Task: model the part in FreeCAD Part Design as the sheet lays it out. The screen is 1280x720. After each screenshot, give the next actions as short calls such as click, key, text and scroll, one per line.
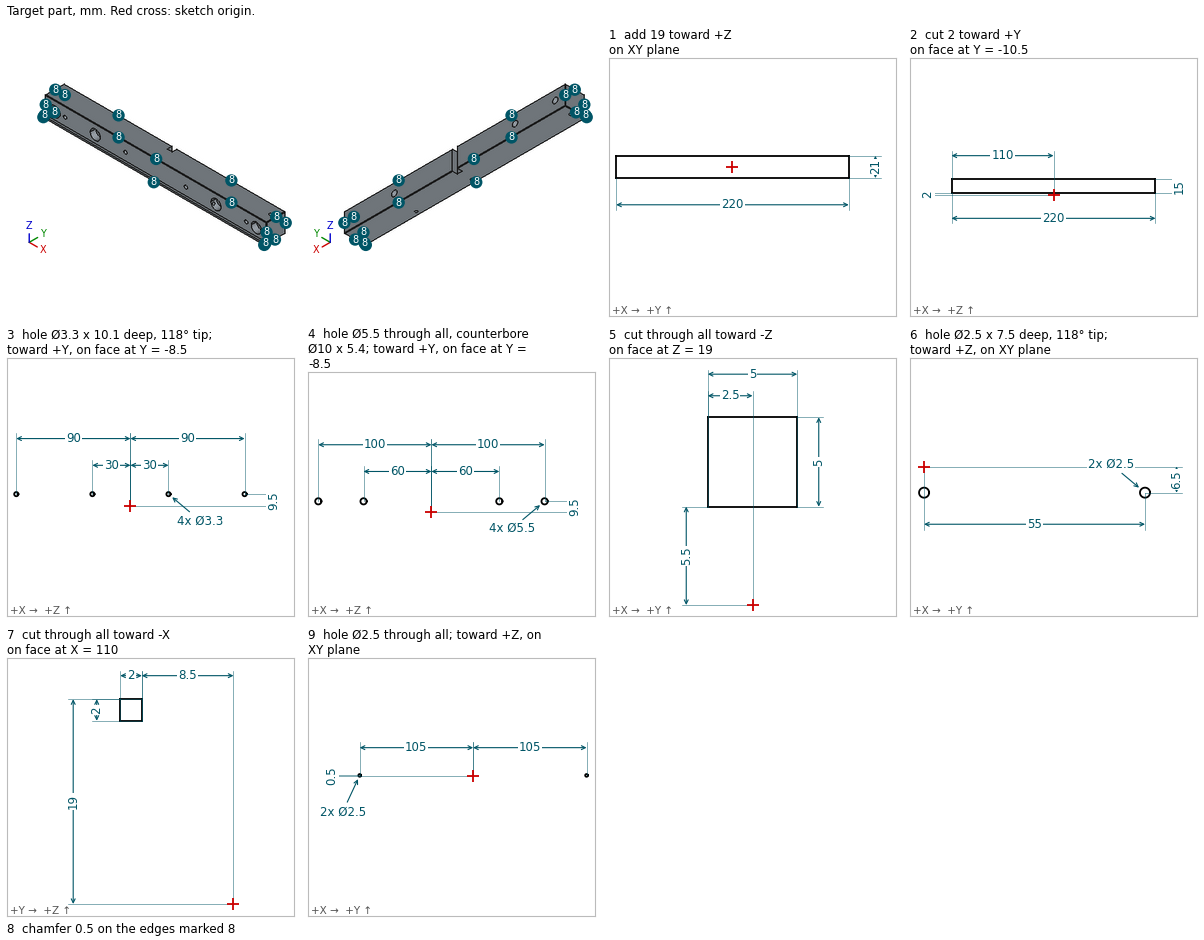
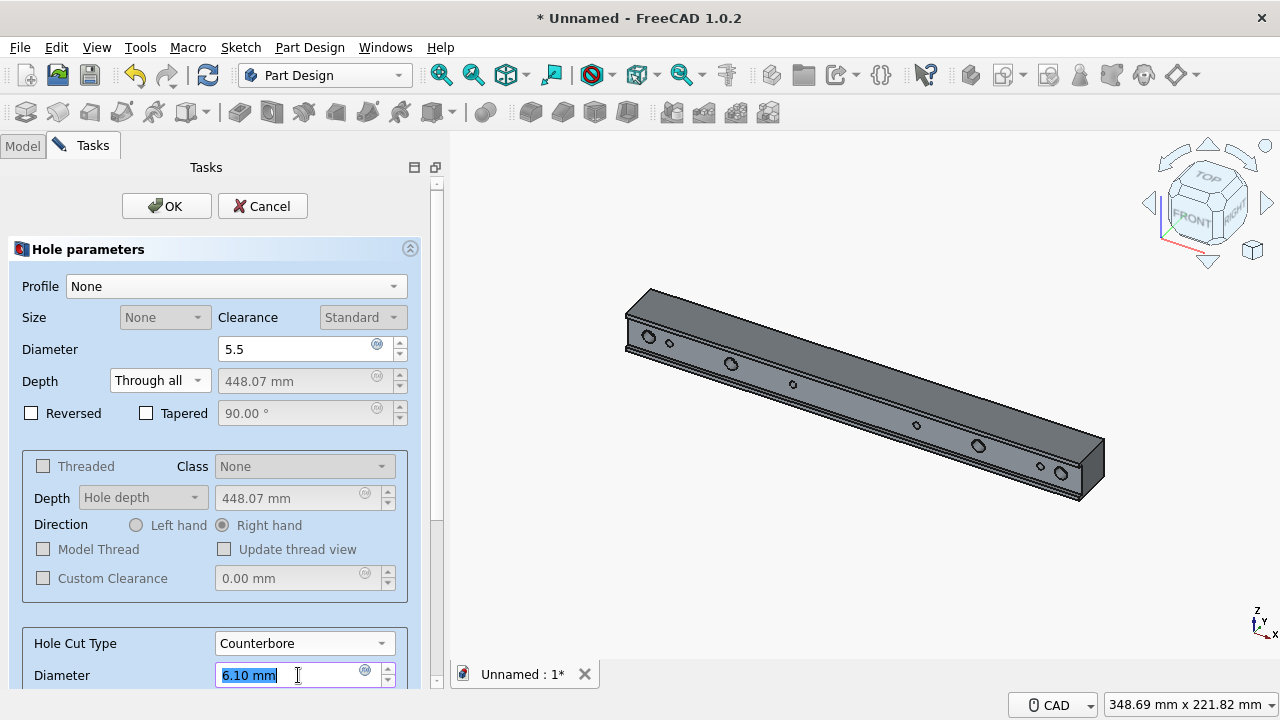
text(10)
key(Tab)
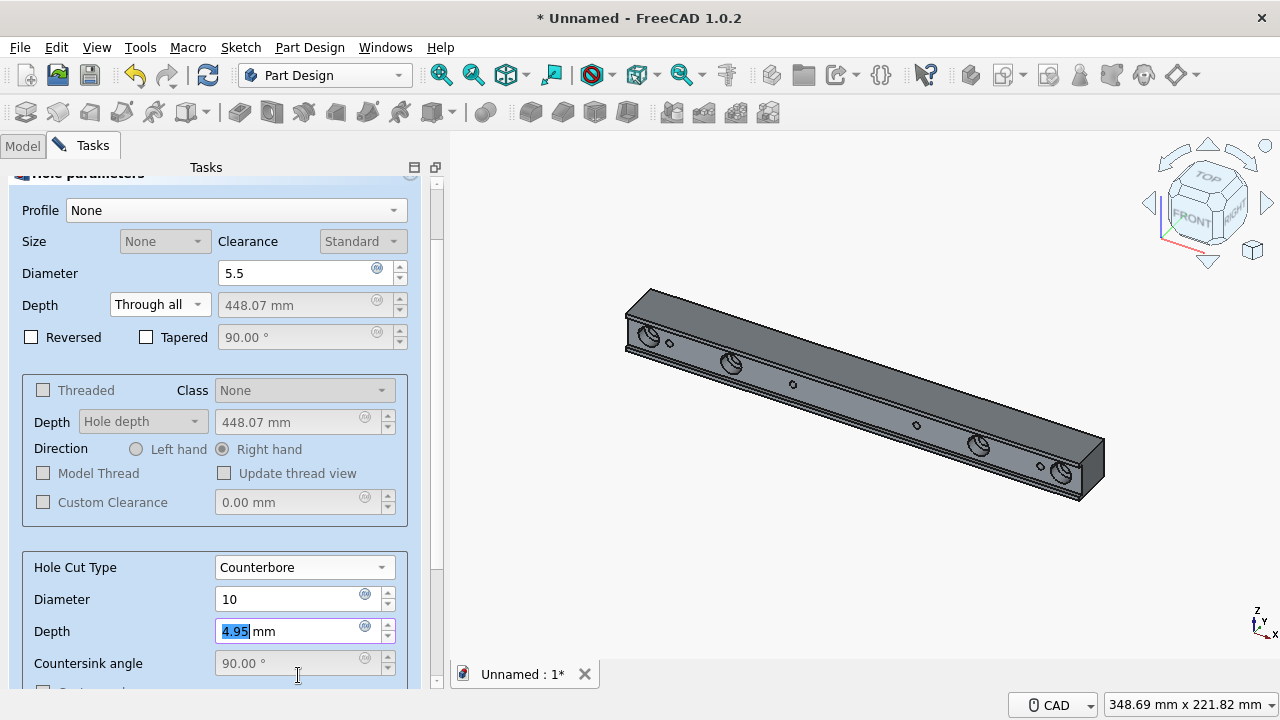
text(5.4)
key(Tab)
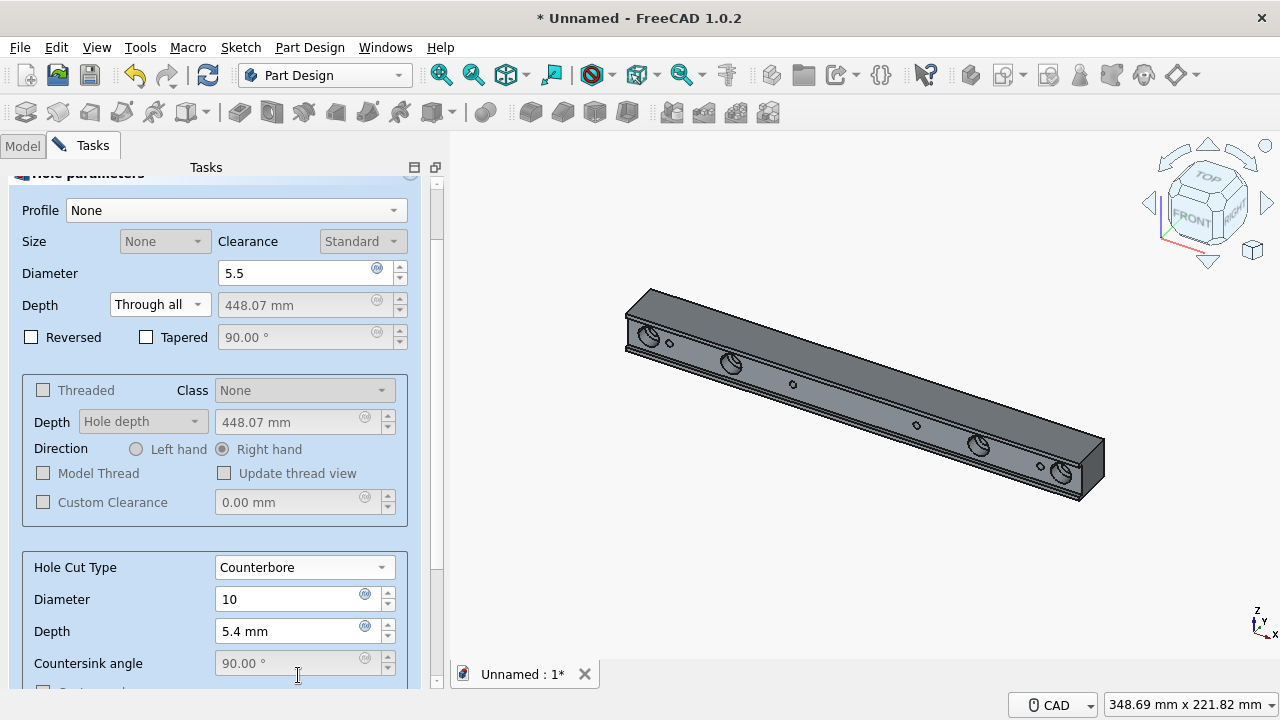
scroll(437, 432, up, 3)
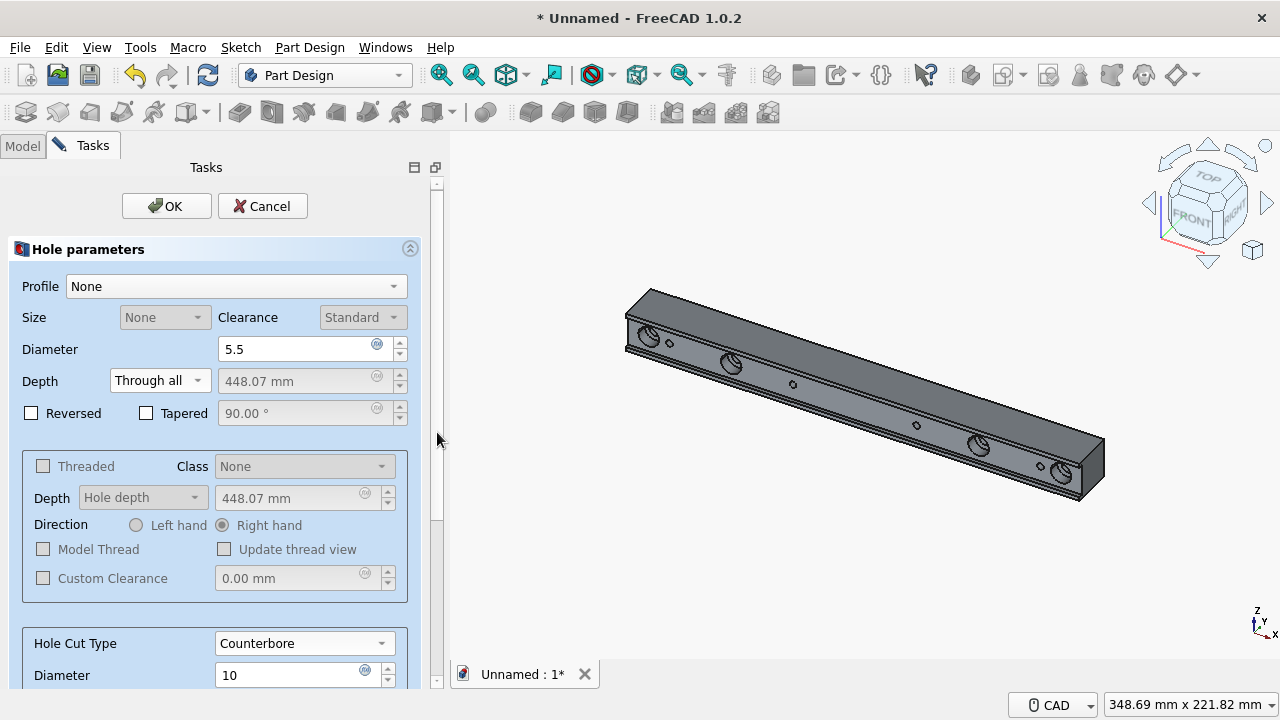
click(167, 206)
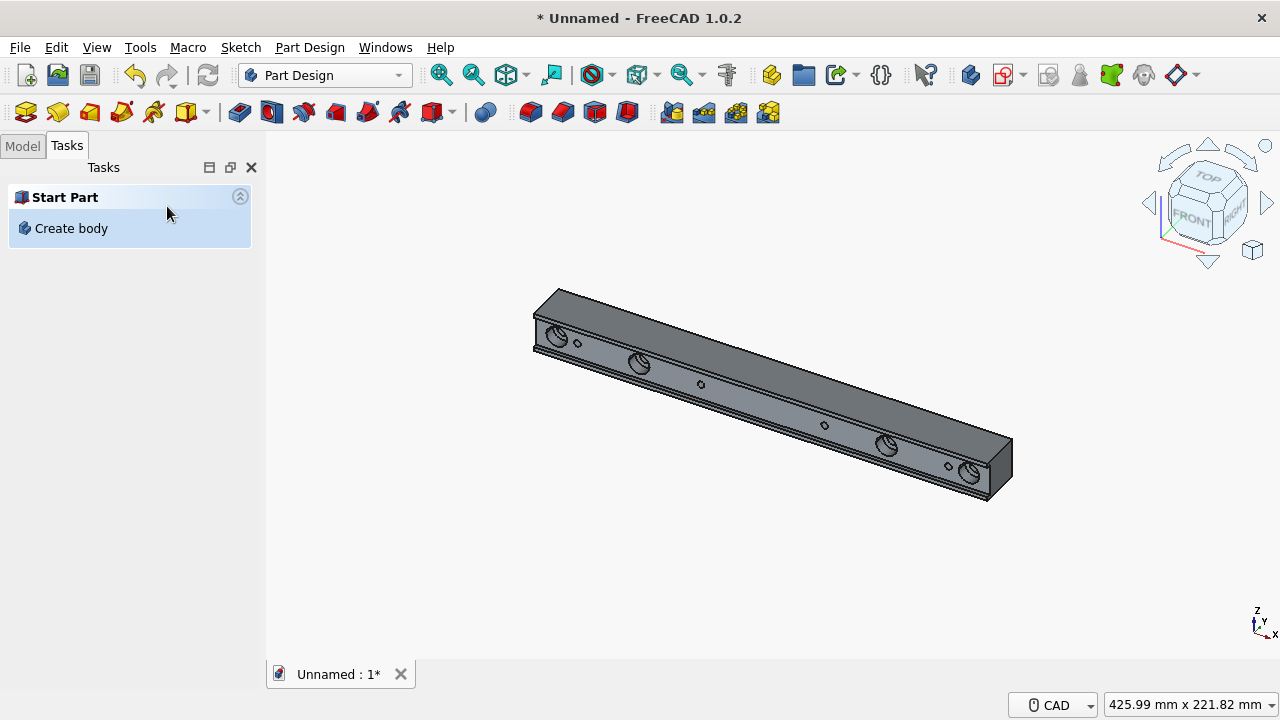
click(967, 440)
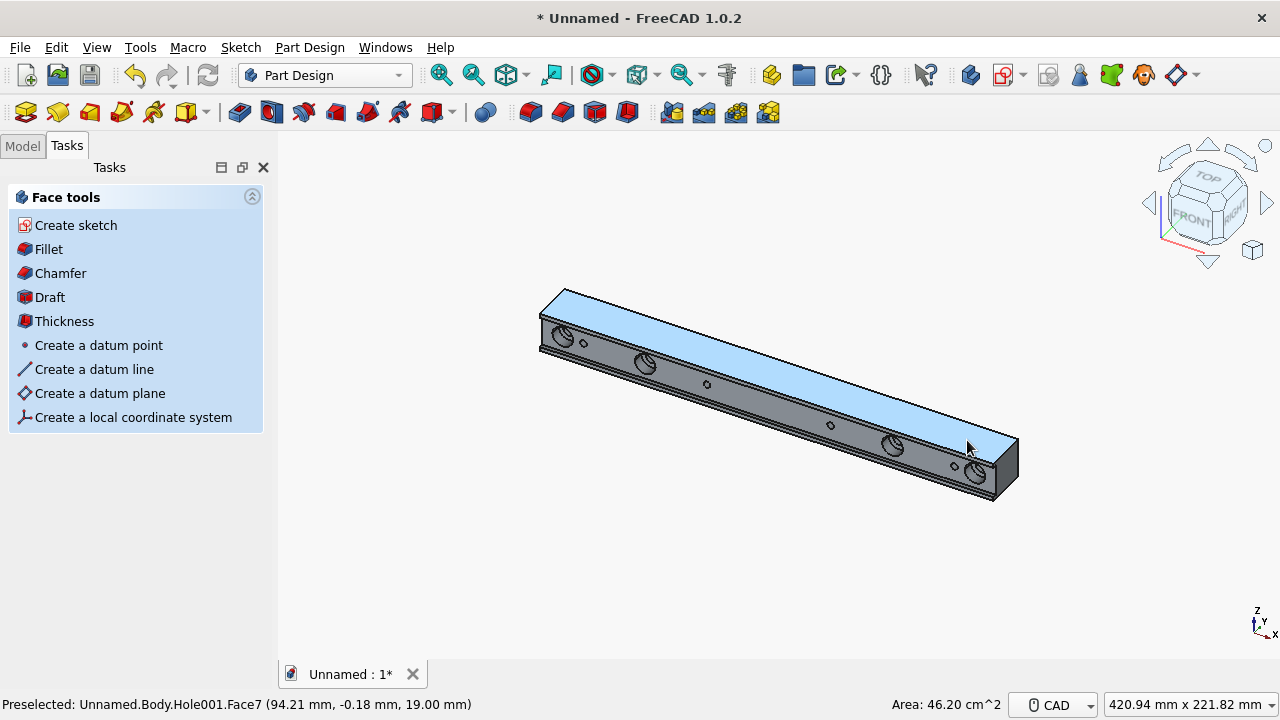
click(1004, 76)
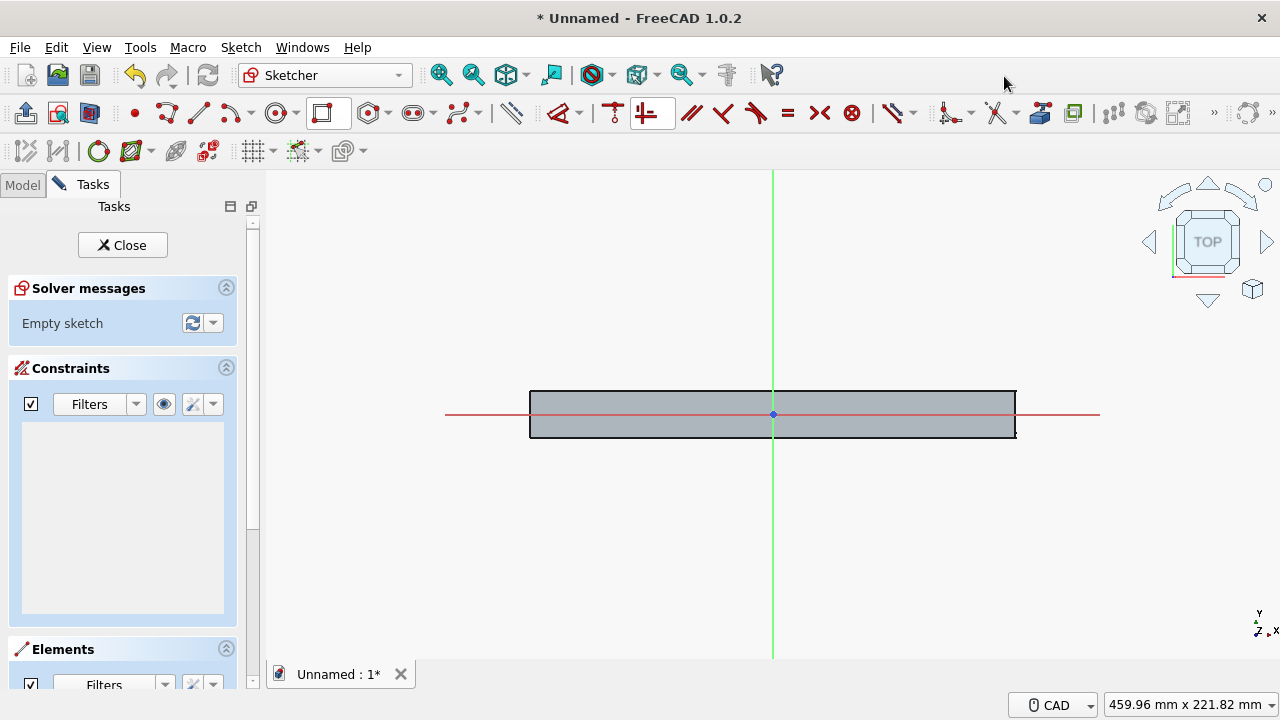
scroll(778, 402, up, 13)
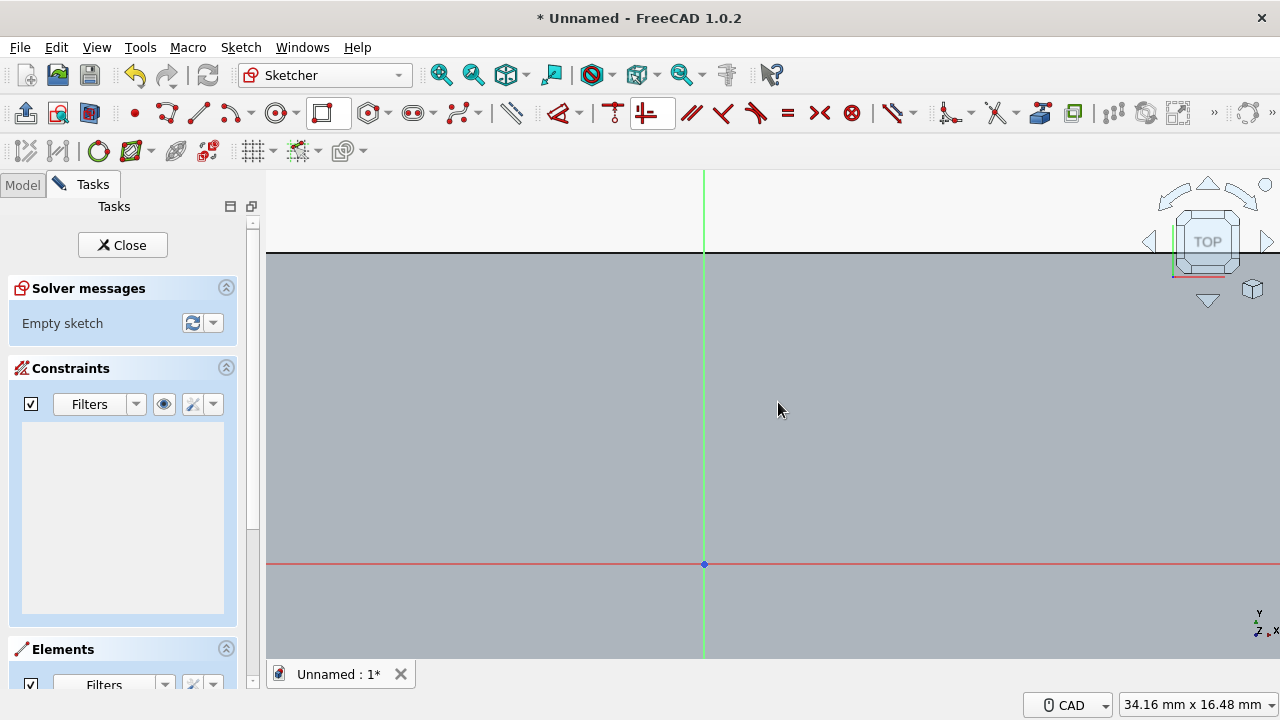
click(322, 114)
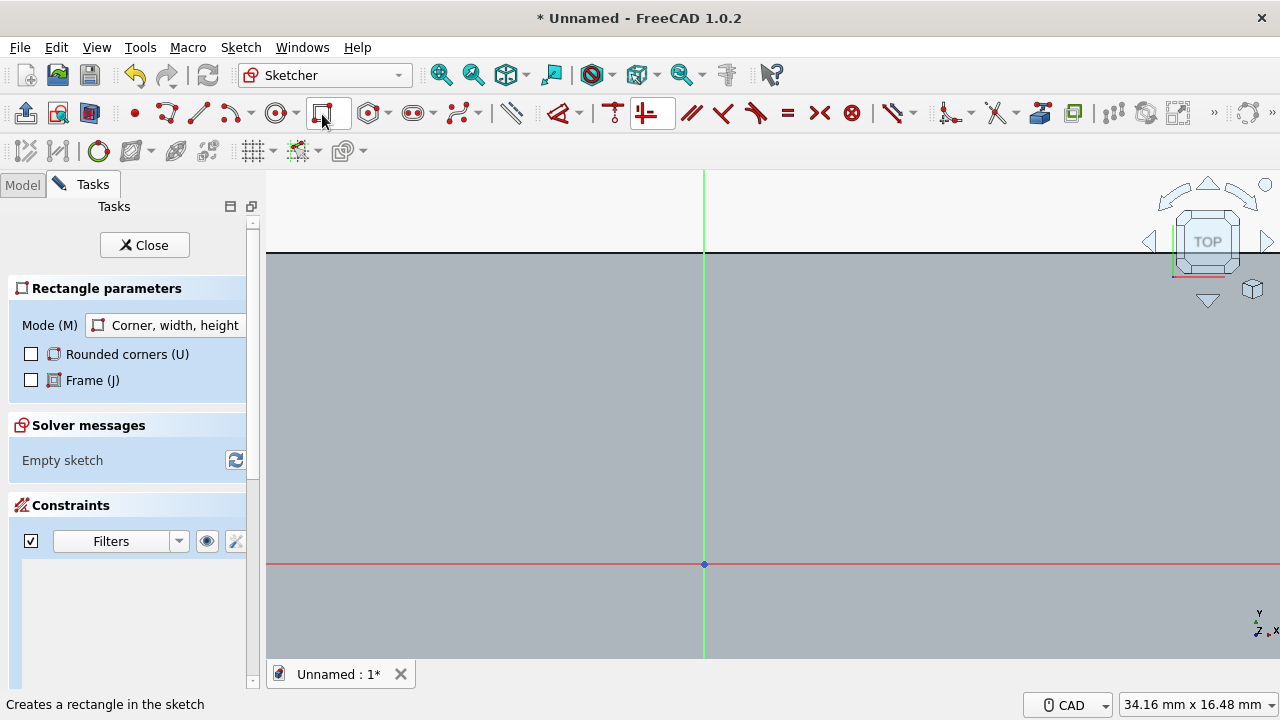
click(630, 253)
move(779, 401)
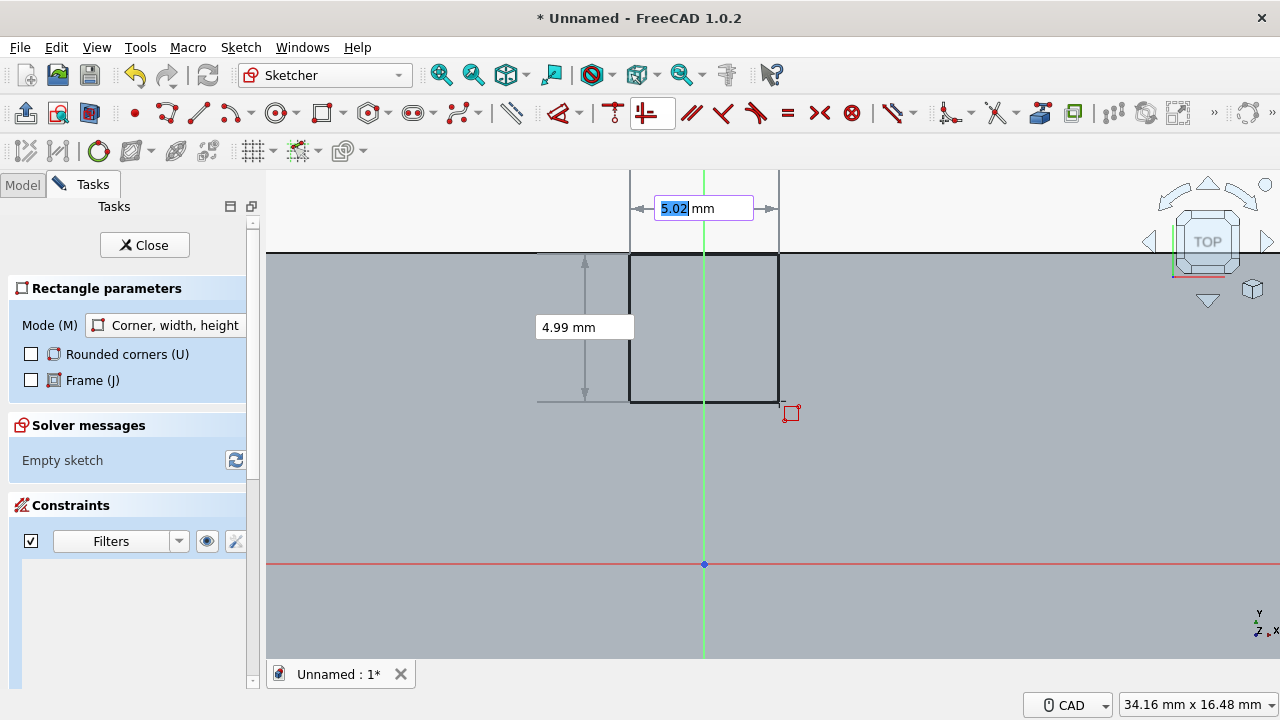
text(5)
key(Tab)
text(5)
key(Return)
key(Escape)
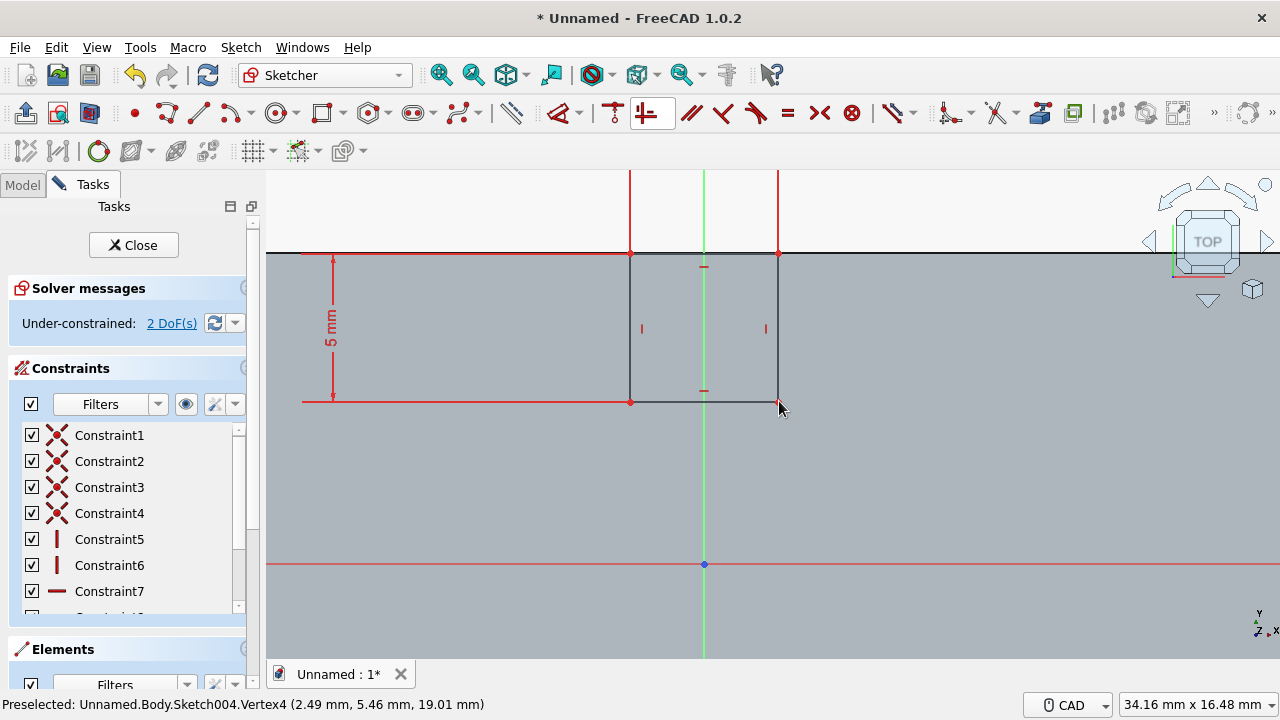
click(558, 114)